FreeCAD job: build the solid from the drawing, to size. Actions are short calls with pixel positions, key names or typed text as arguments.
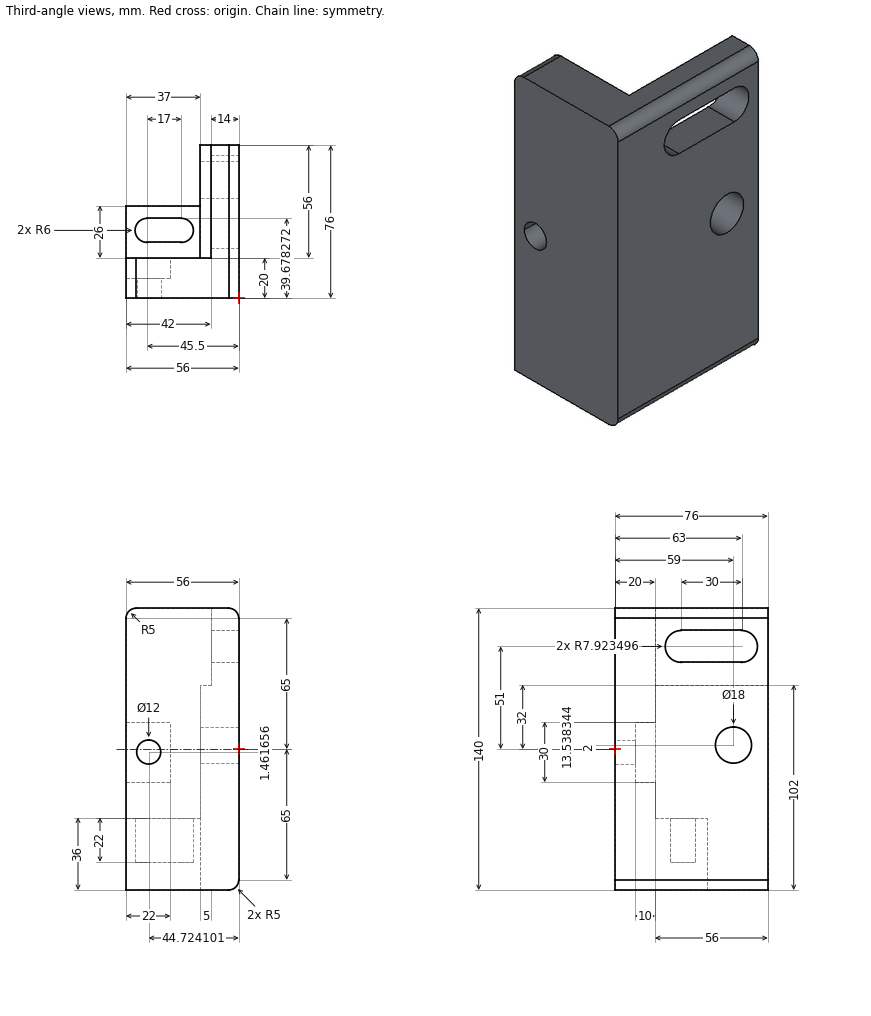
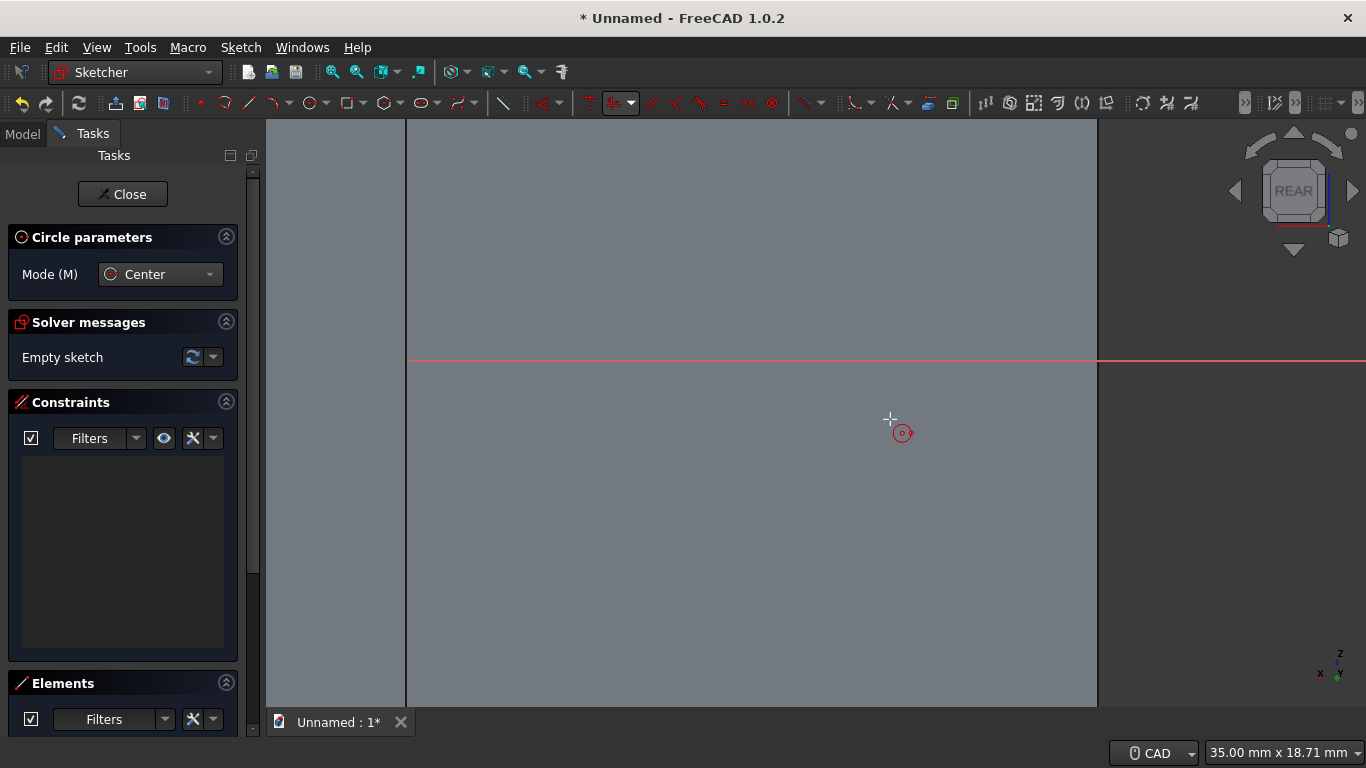
click(743, 407)
click(877, 273)
key(Escape)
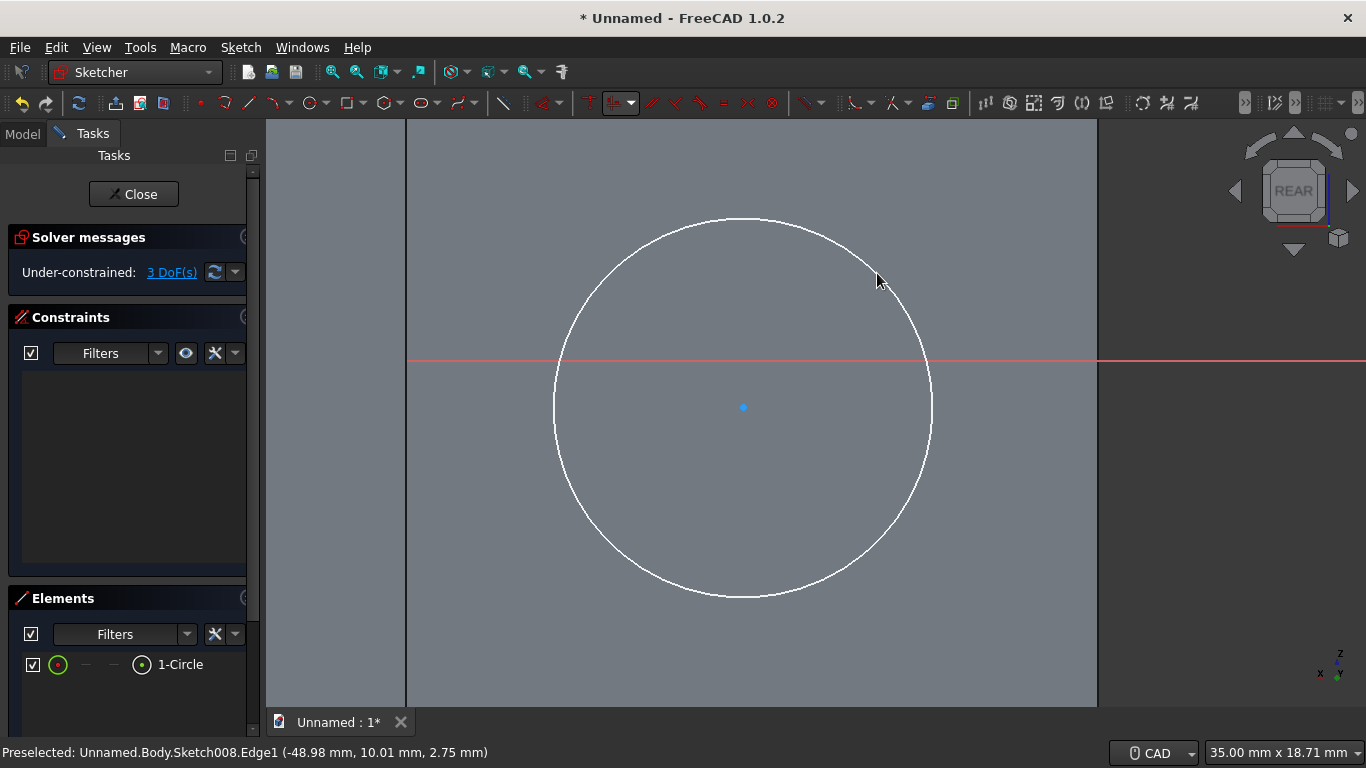
click(542, 104)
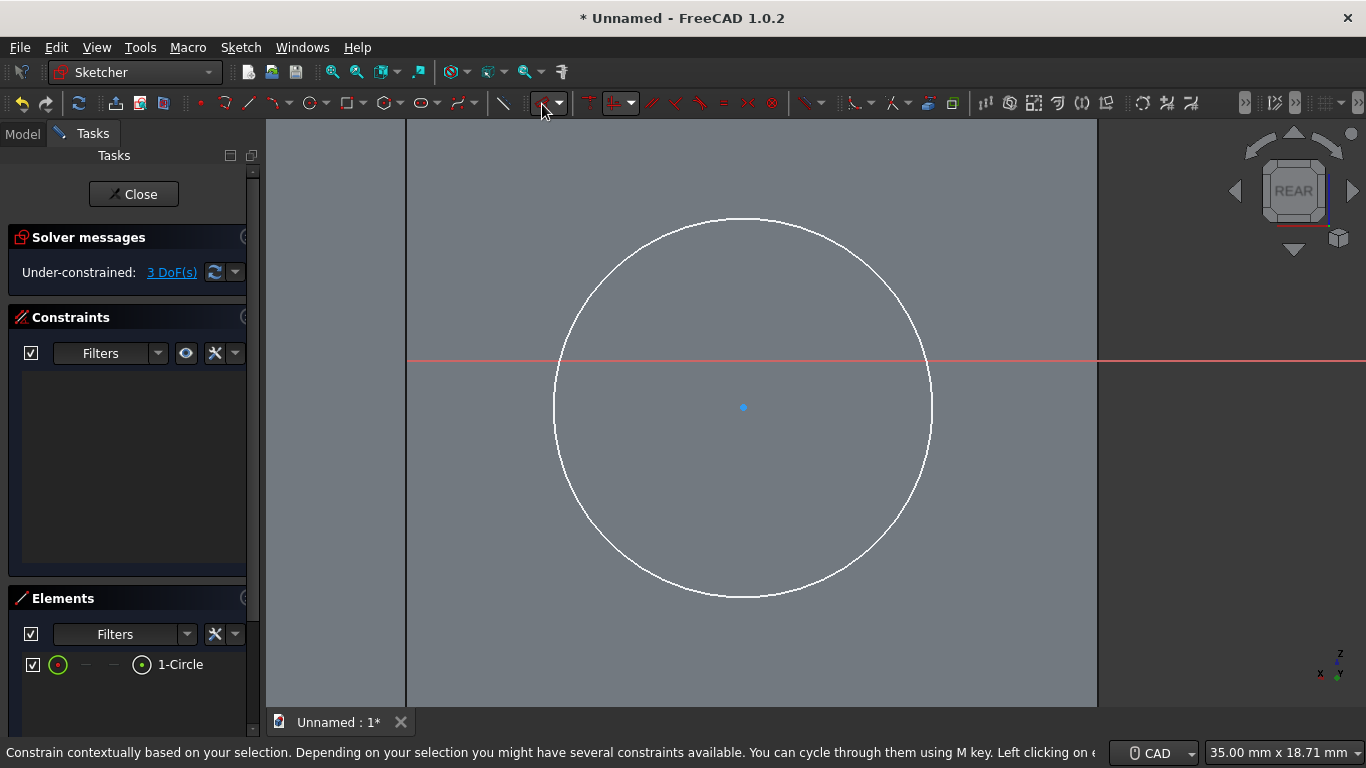
click(877, 274)
click(900, 251)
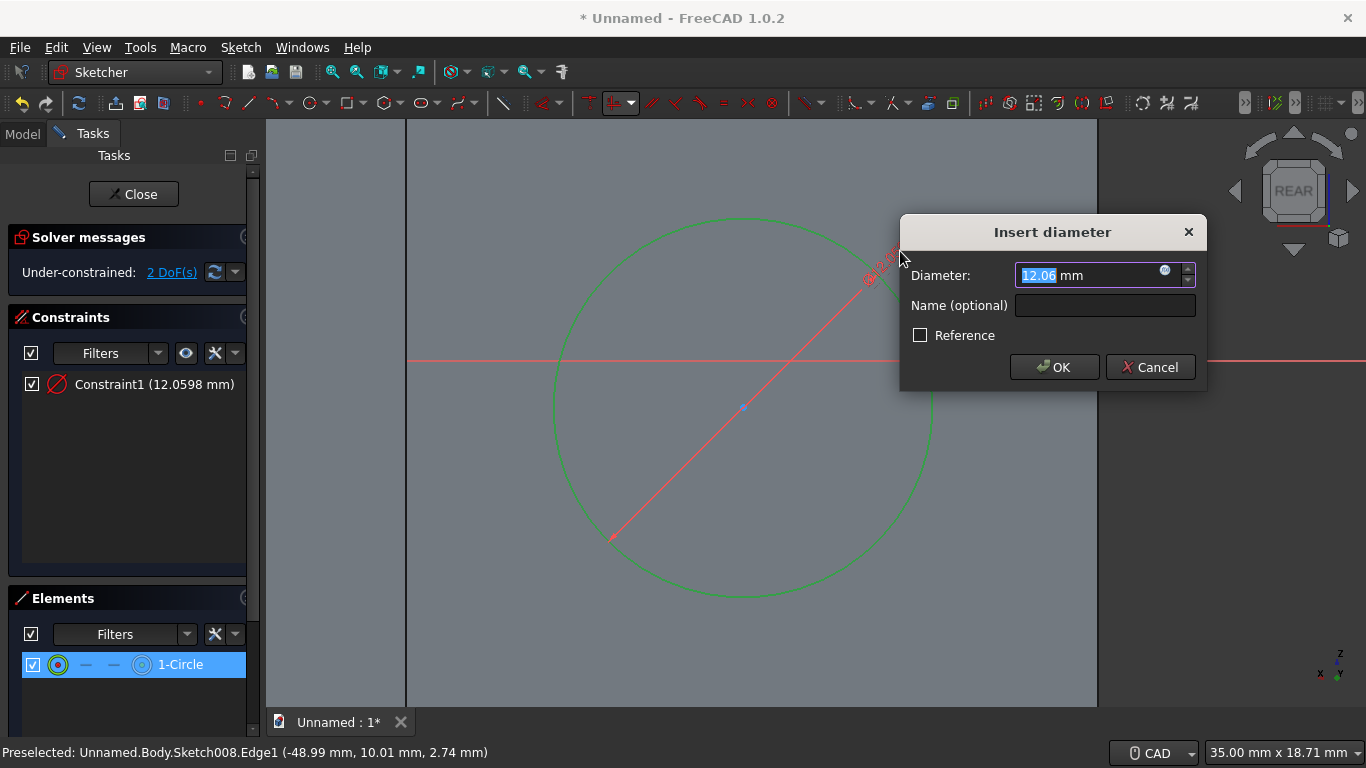
text(12)
key(Return)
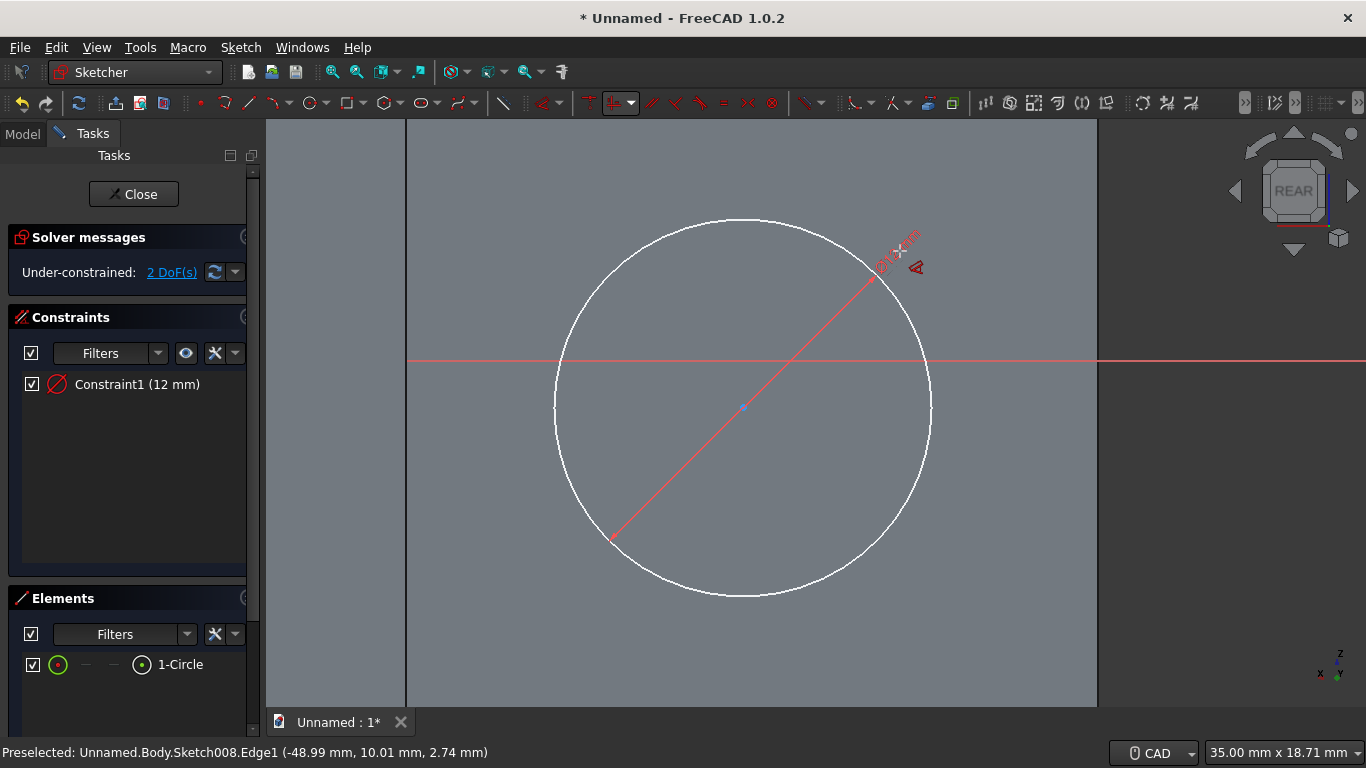
click(743, 408)
click(777, 384)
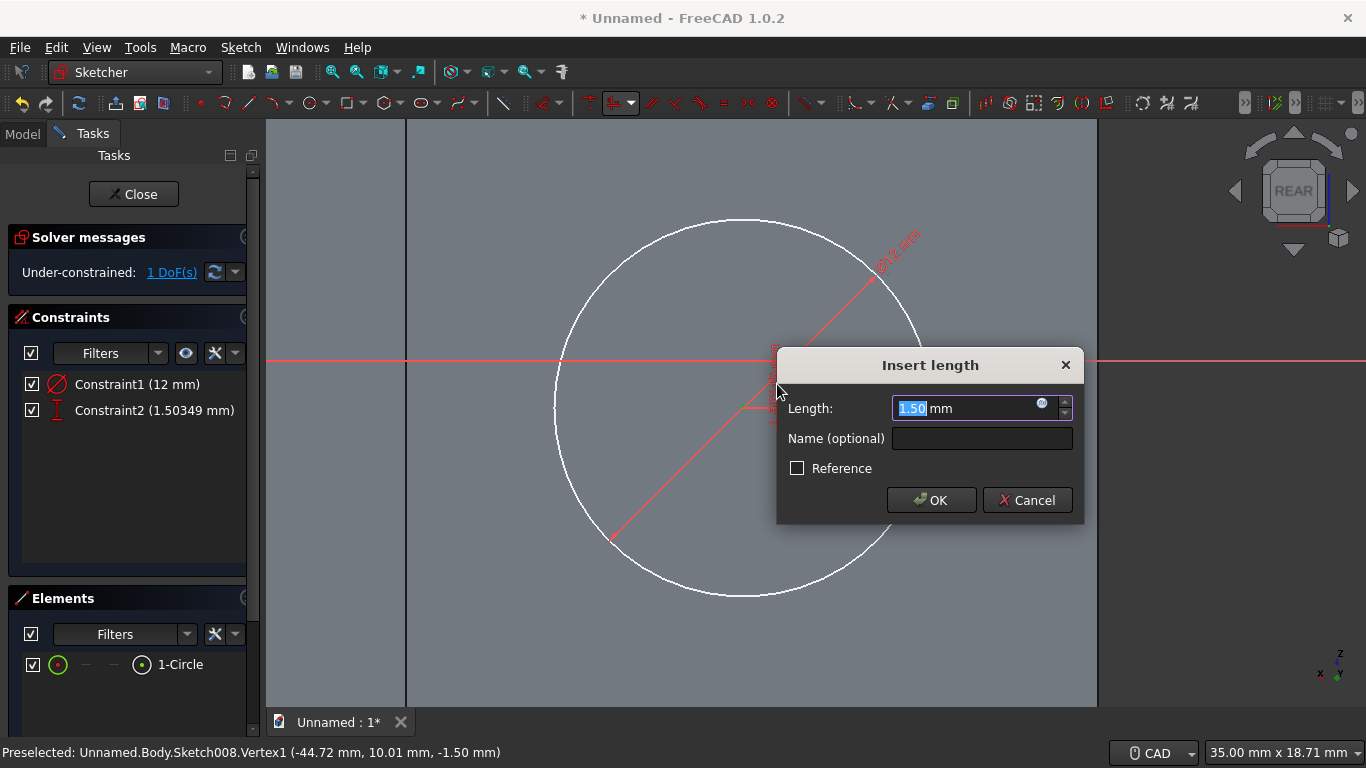
text(1.461656)
key(Return)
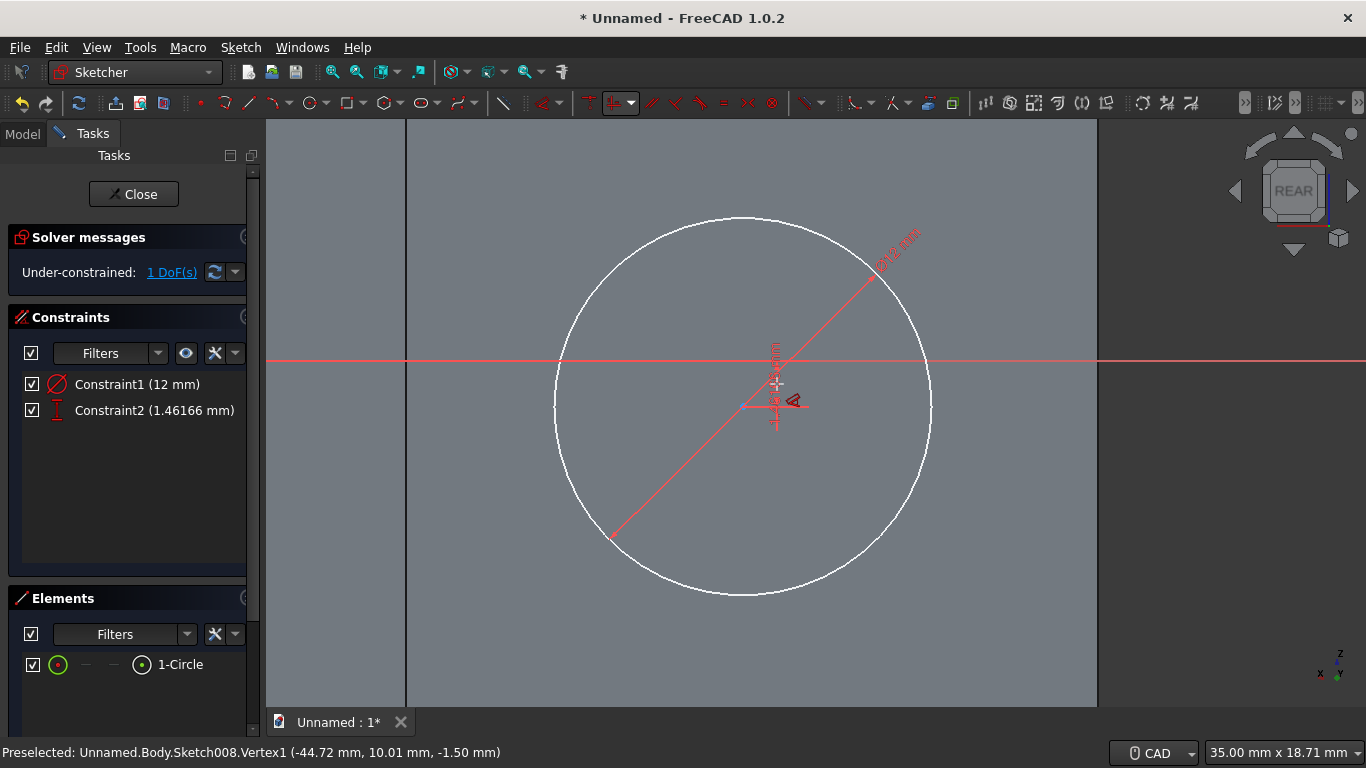
click(743, 407)
click(518, 327)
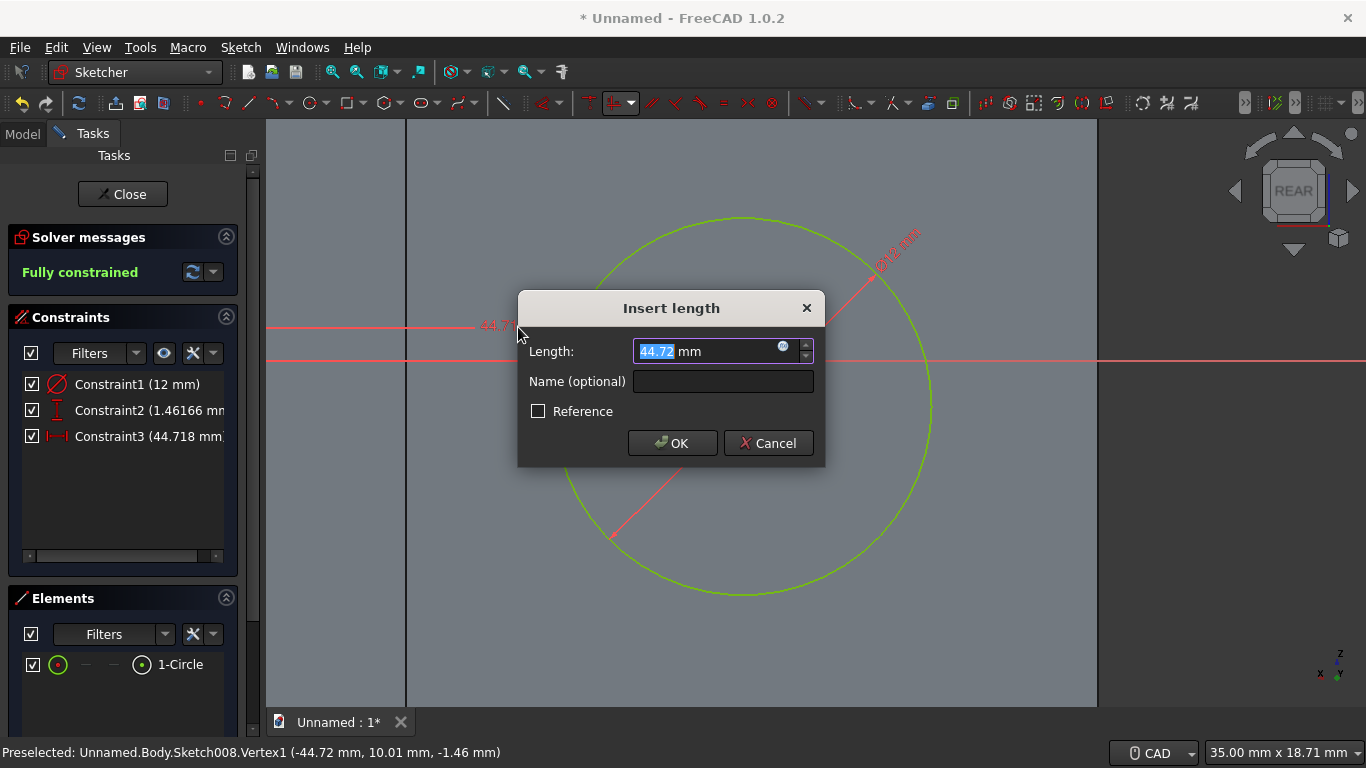
text(44.724101)
key(Return)
key(Escape)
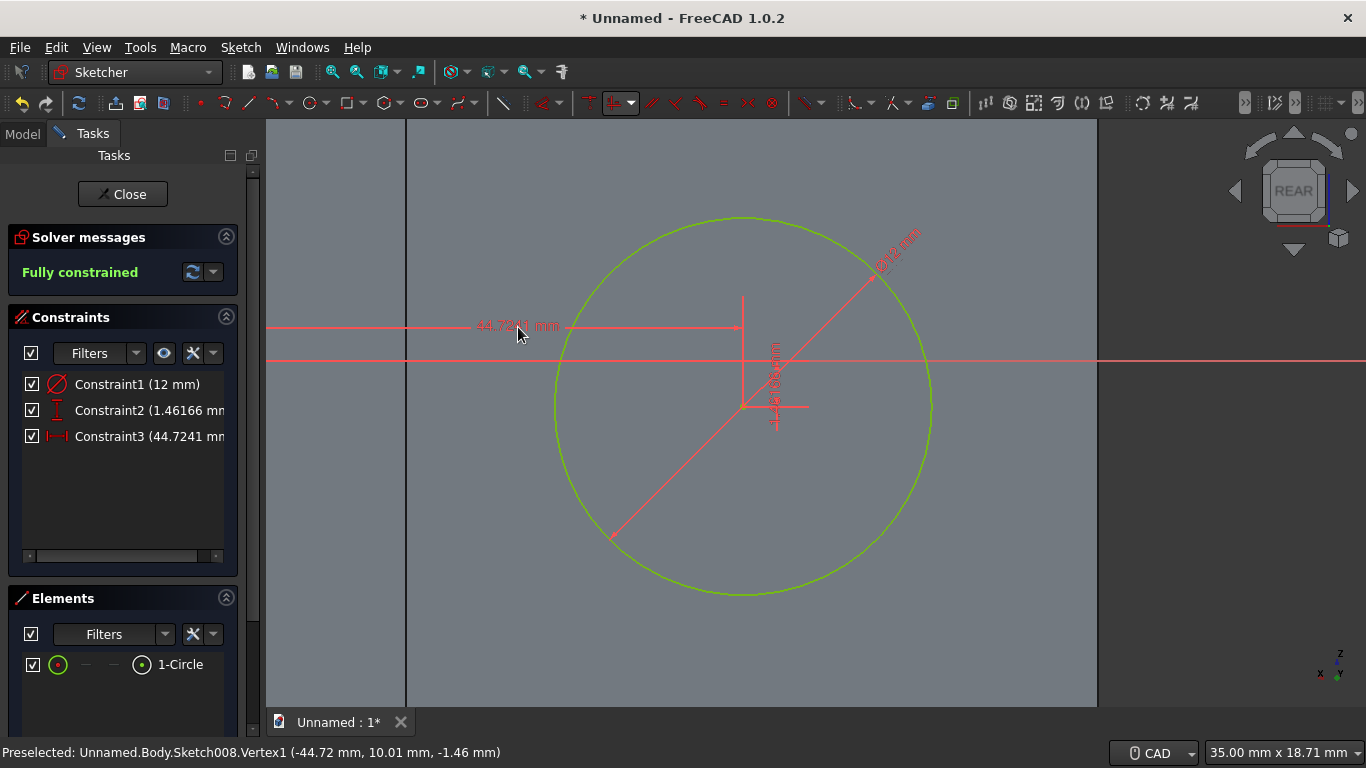
click(123, 194)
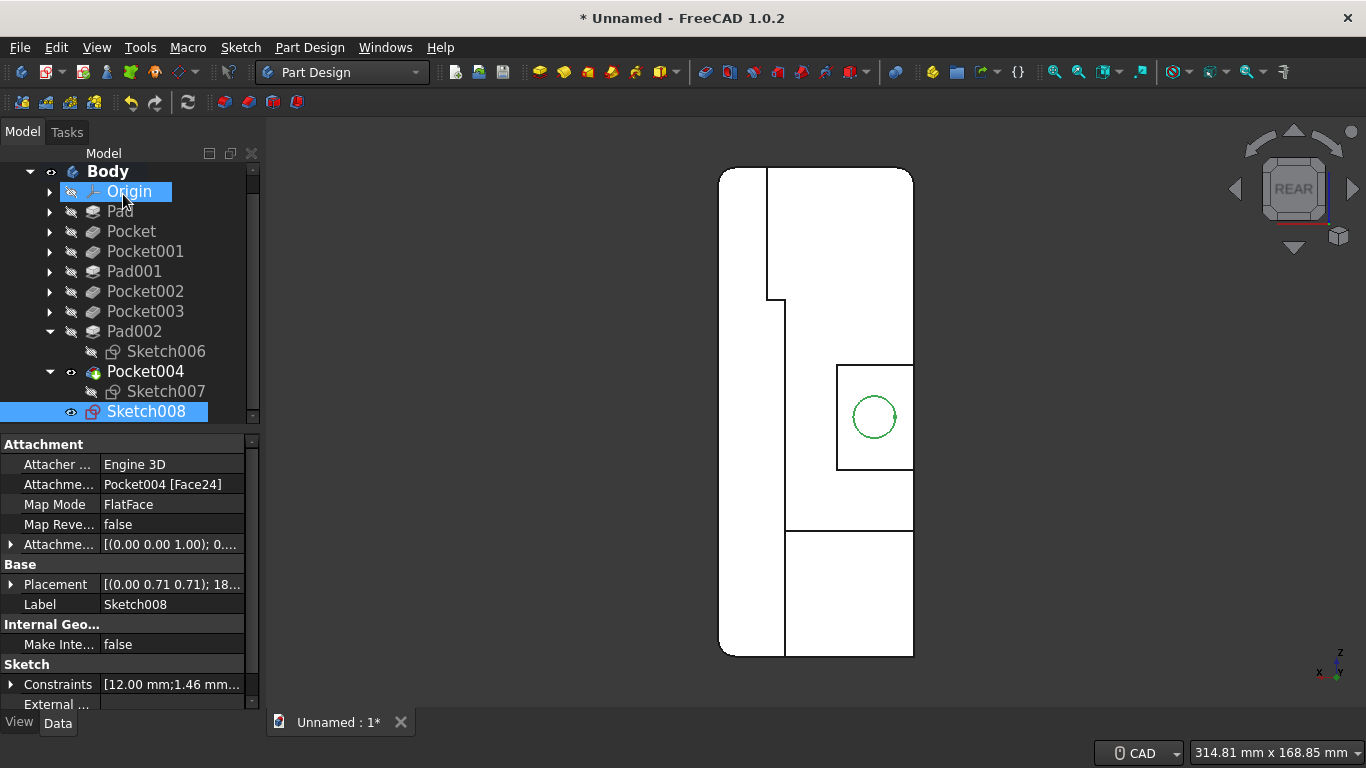
click(706, 72)